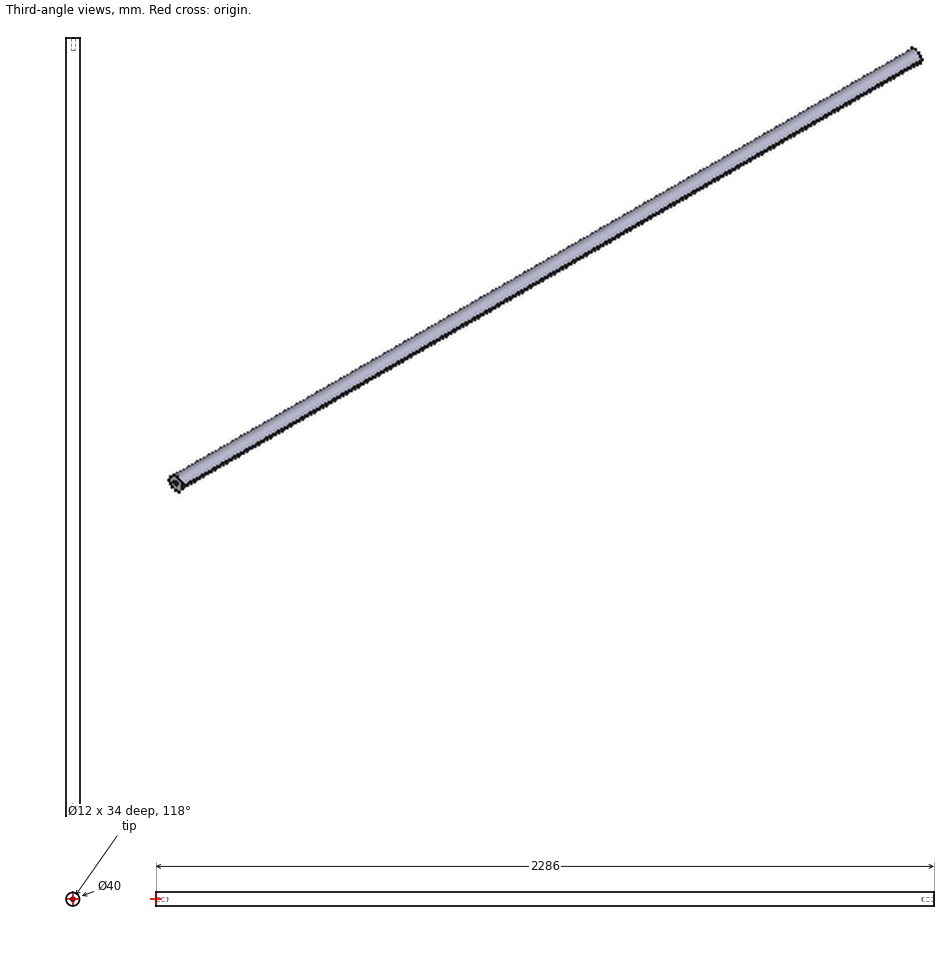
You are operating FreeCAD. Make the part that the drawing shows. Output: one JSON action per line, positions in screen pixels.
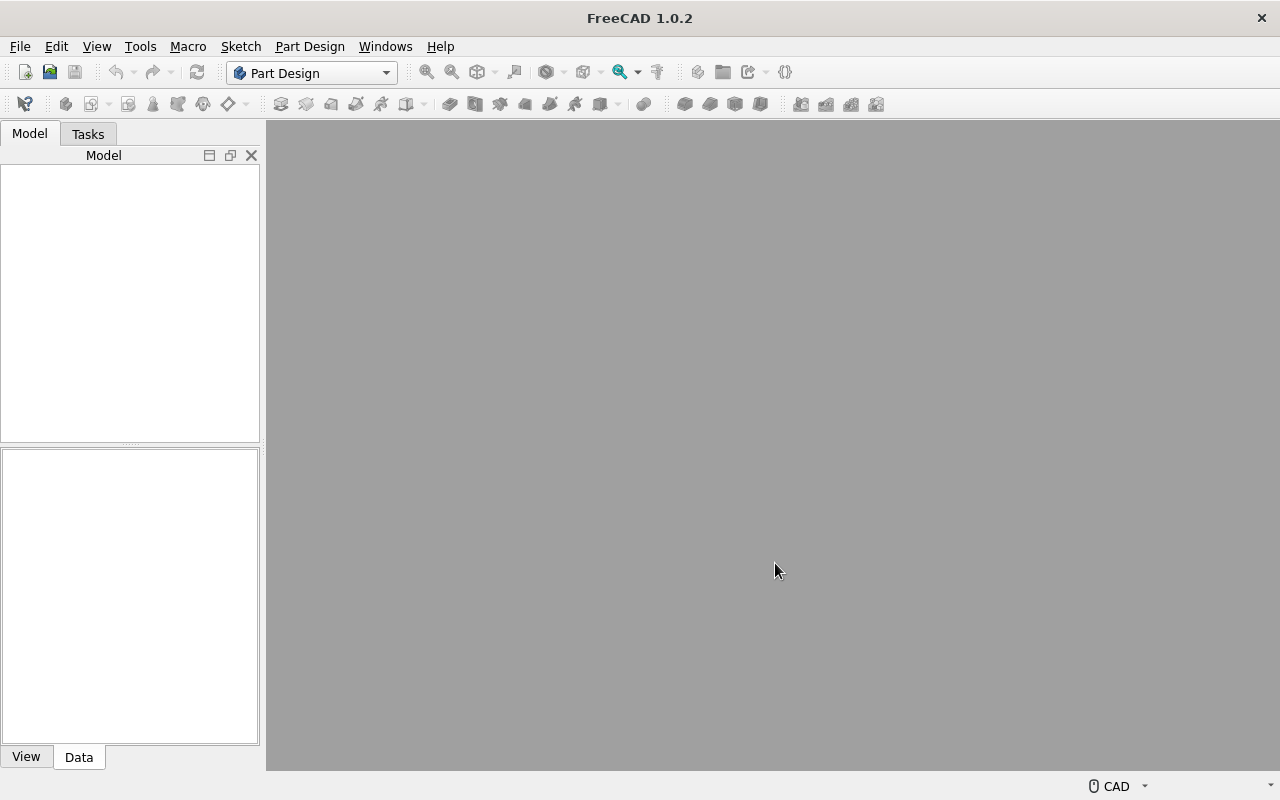
{"action": "left_click", "coordinate": [25, 72]}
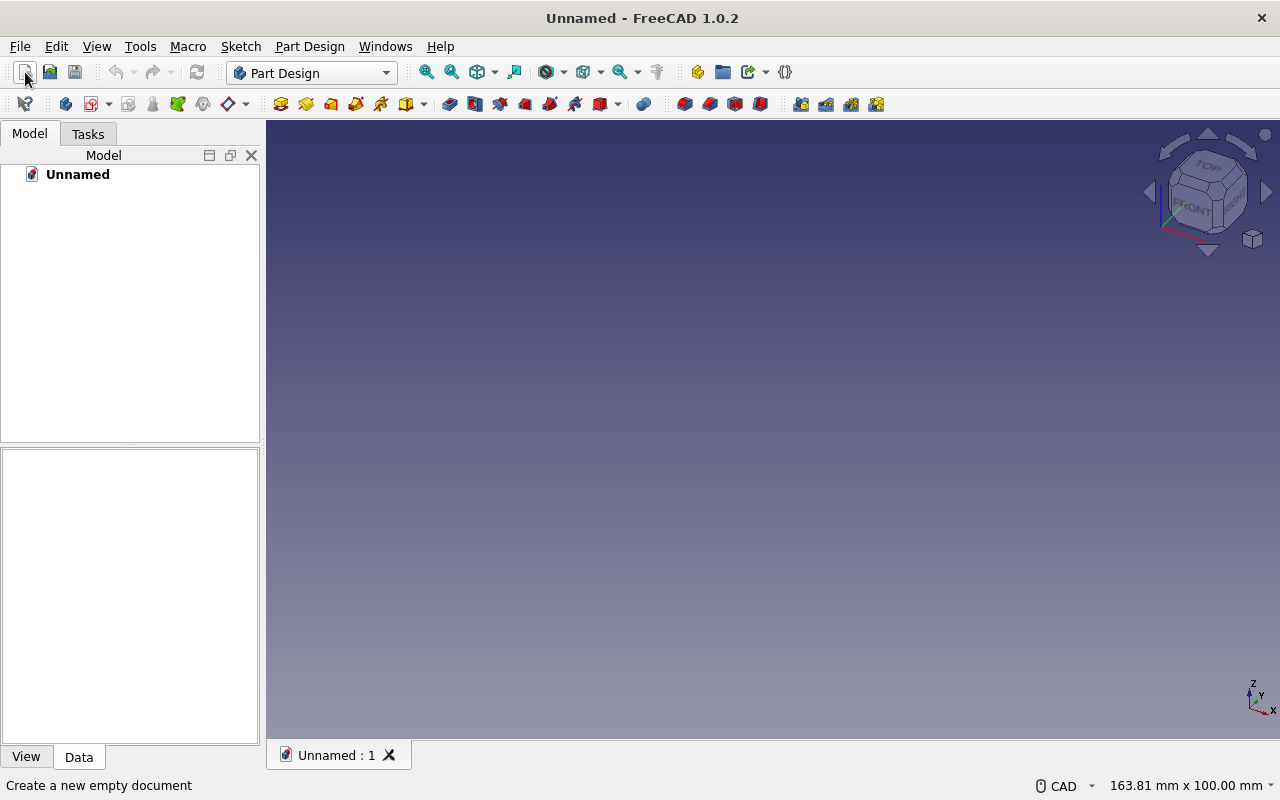
{"action": "left_click", "coordinate": [90, 104]}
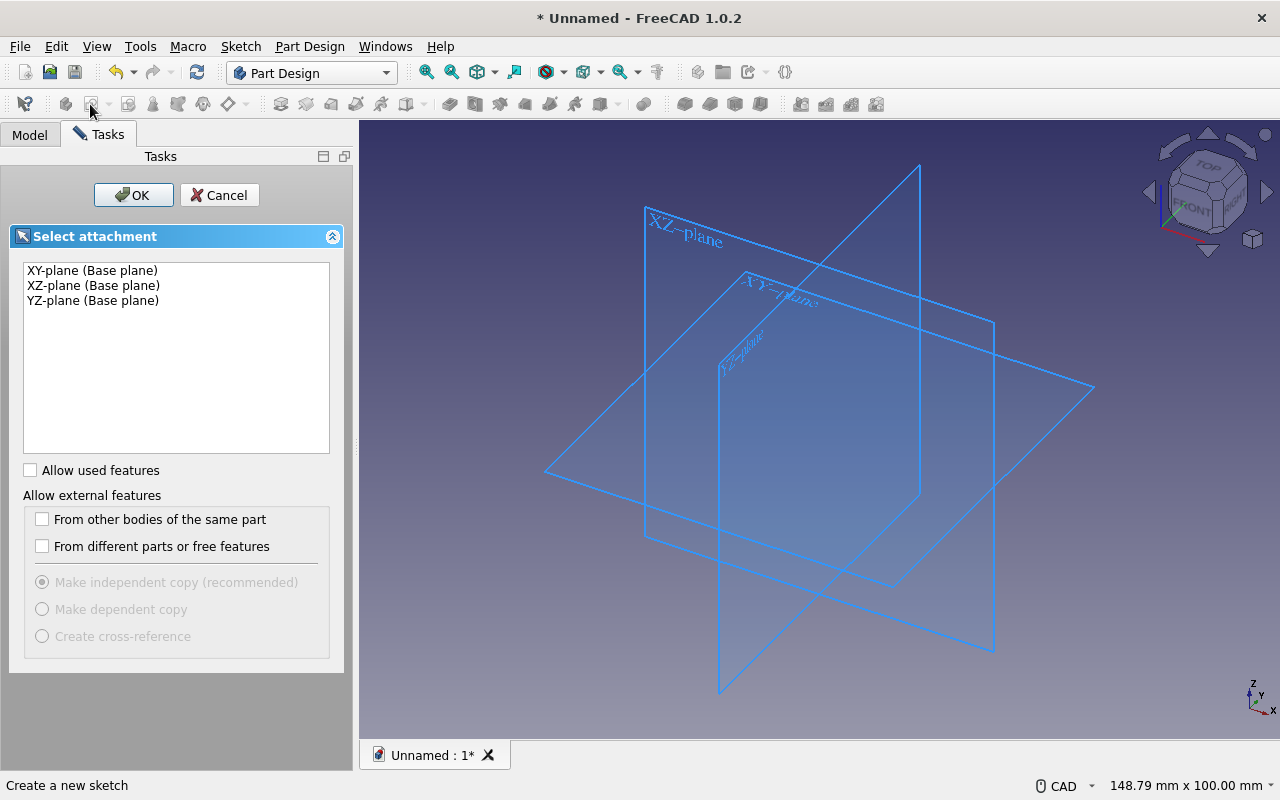
{"action": "left_click", "coordinate": [84, 286]}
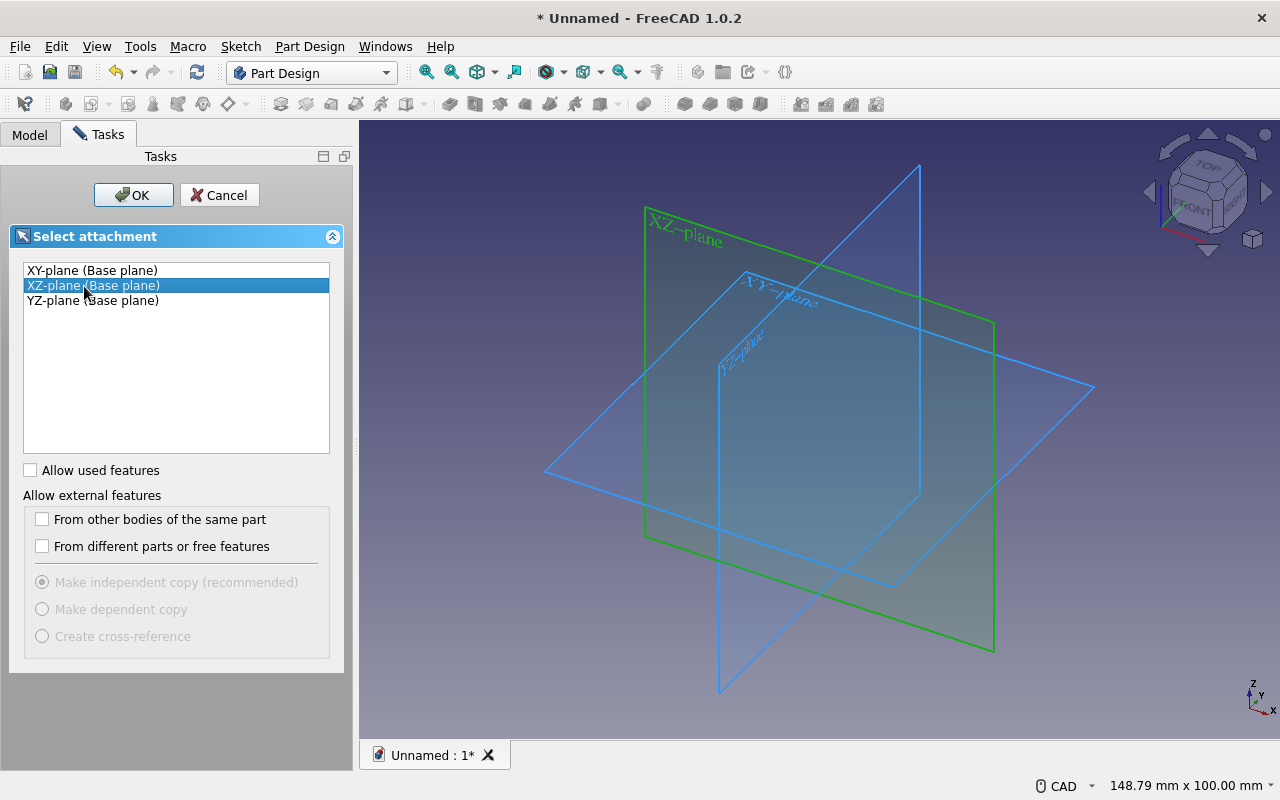
{"action": "left_click", "coordinate": [134, 195]}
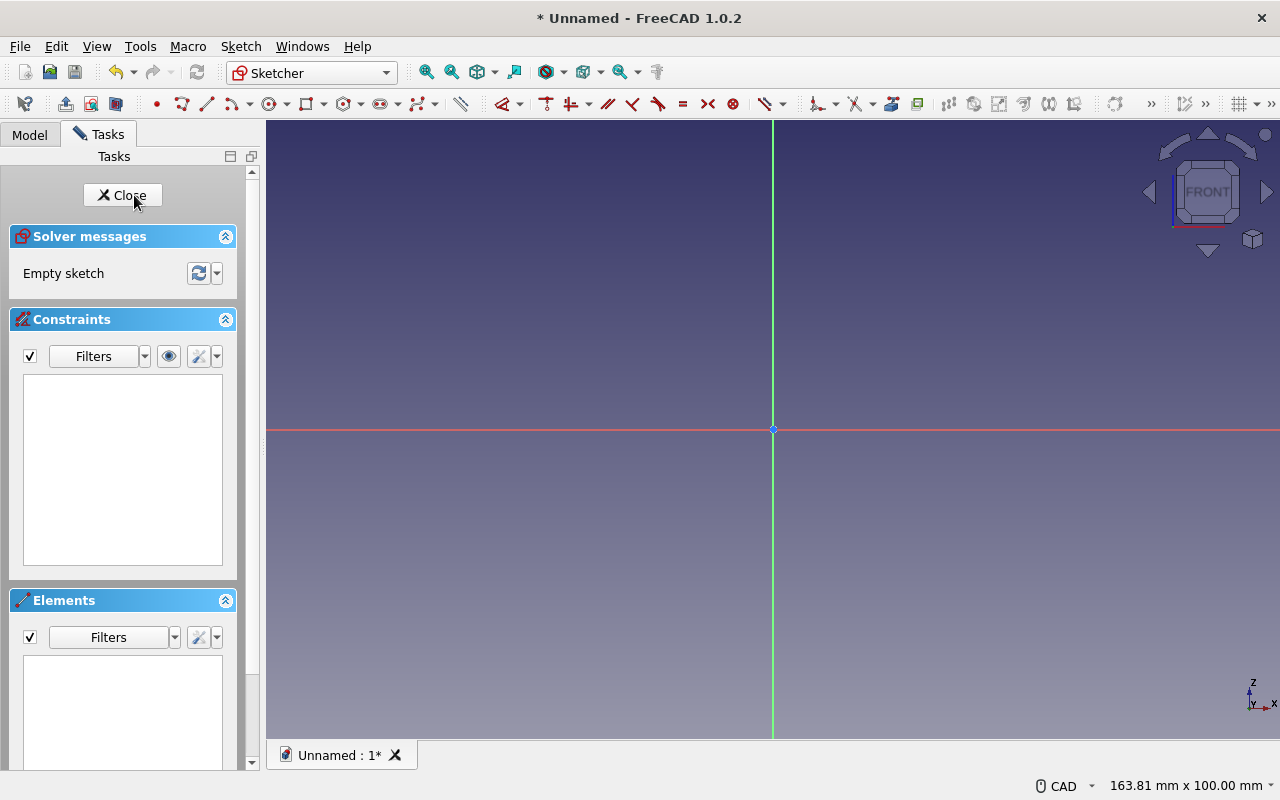
{"action": "scroll", "coordinate": [912, 429], "scroll_direction": "up", "scroll_amount": 2}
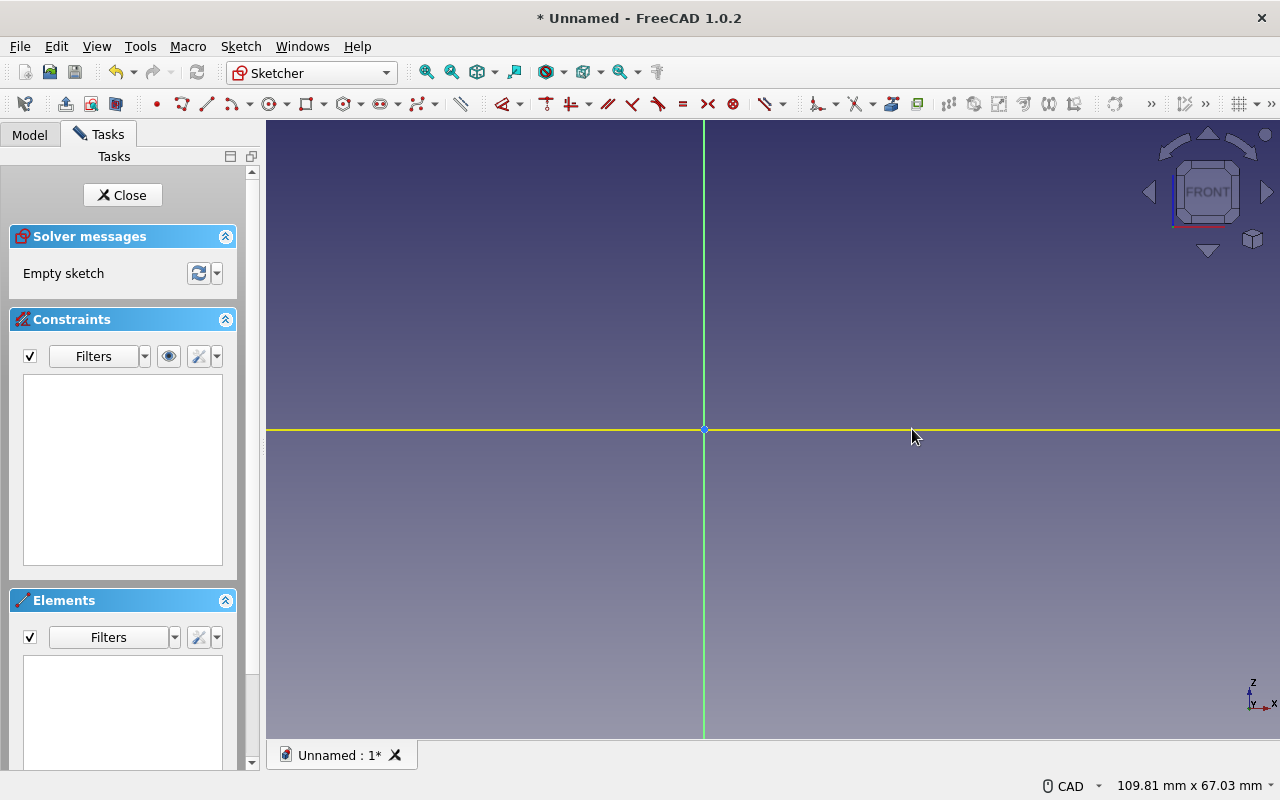
{"action": "left_click", "coordinate": [268, 104]}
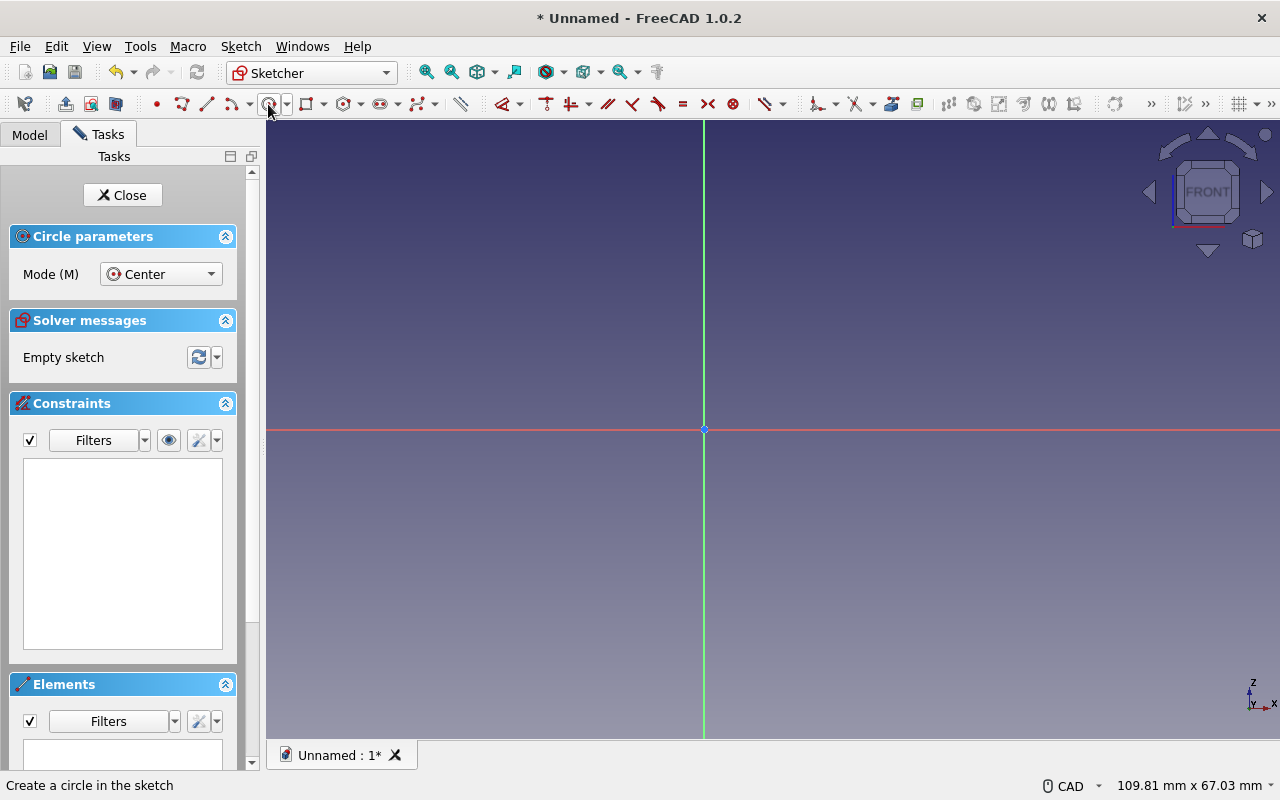
{"action": "left_click", "coordinate": [704, 430]}
{"action": "mouse_move", "coordinate": [835, 299]}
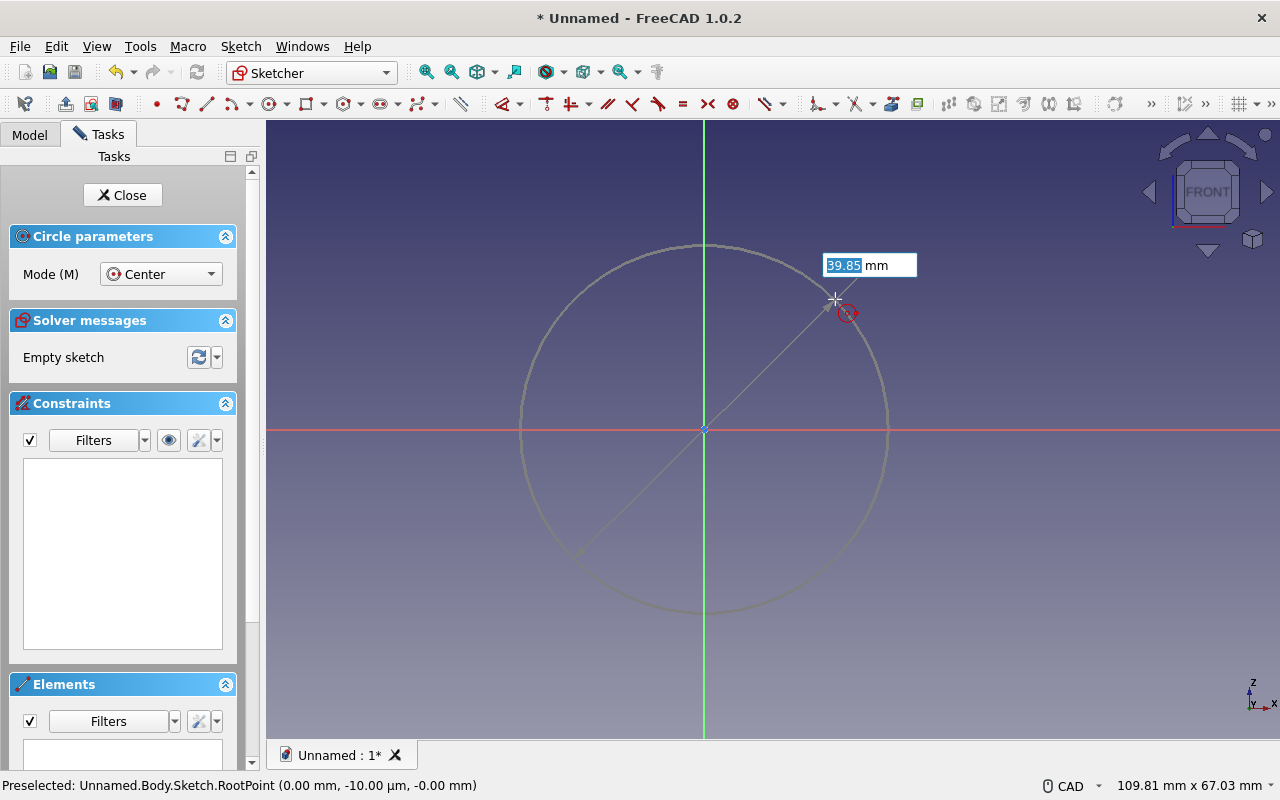
{"action": "type", "text": "40"}
{"action": "key", "text": "Return"}
{"action": "key", "text": "Escape"}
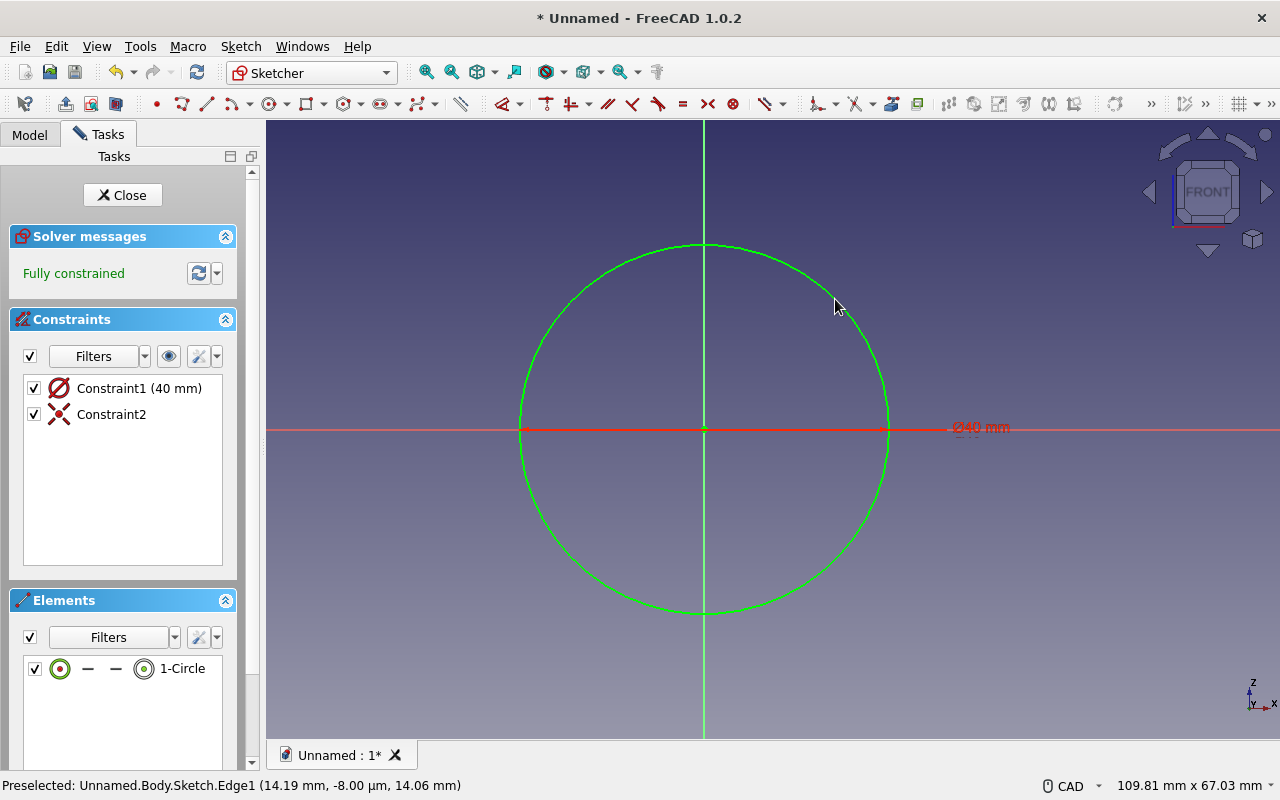
{"action": "left_click", "coordinate": [123, 195]}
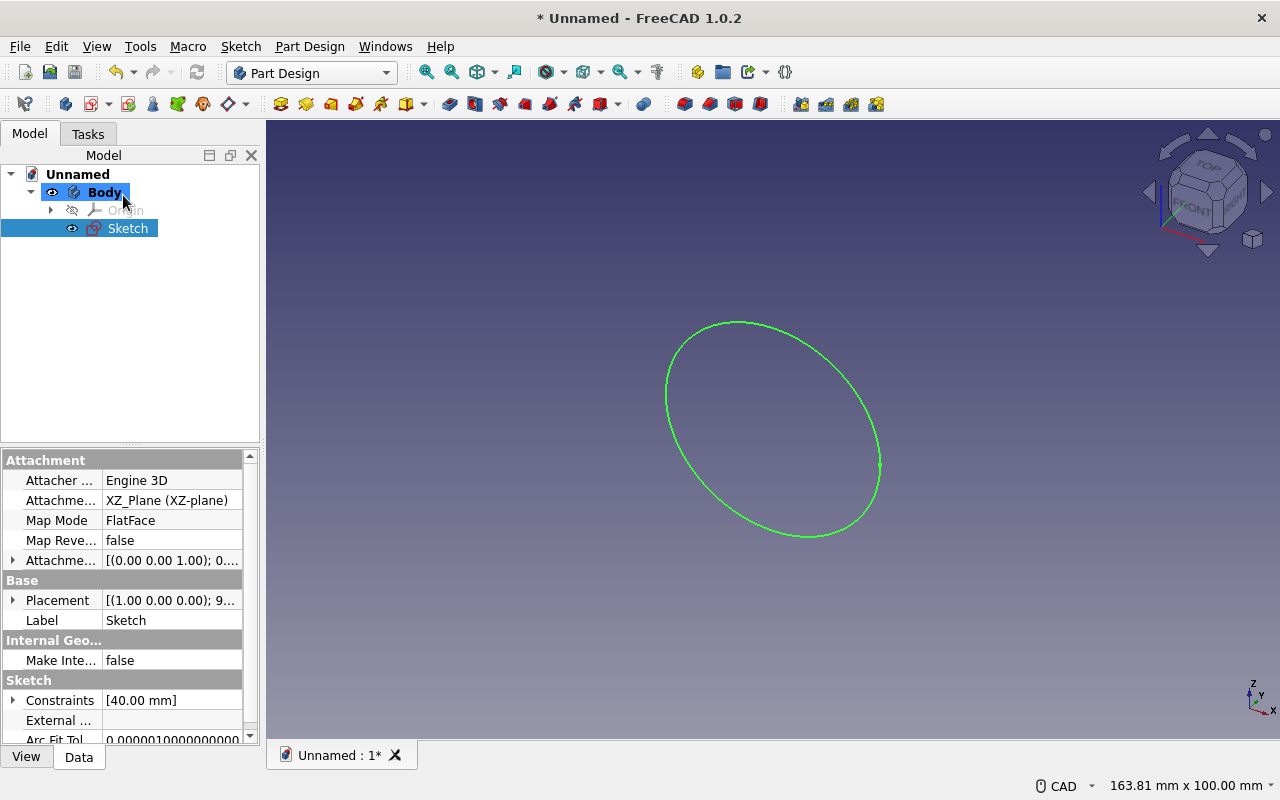
{"action": "left_click", "coordinate": [281, 104]}